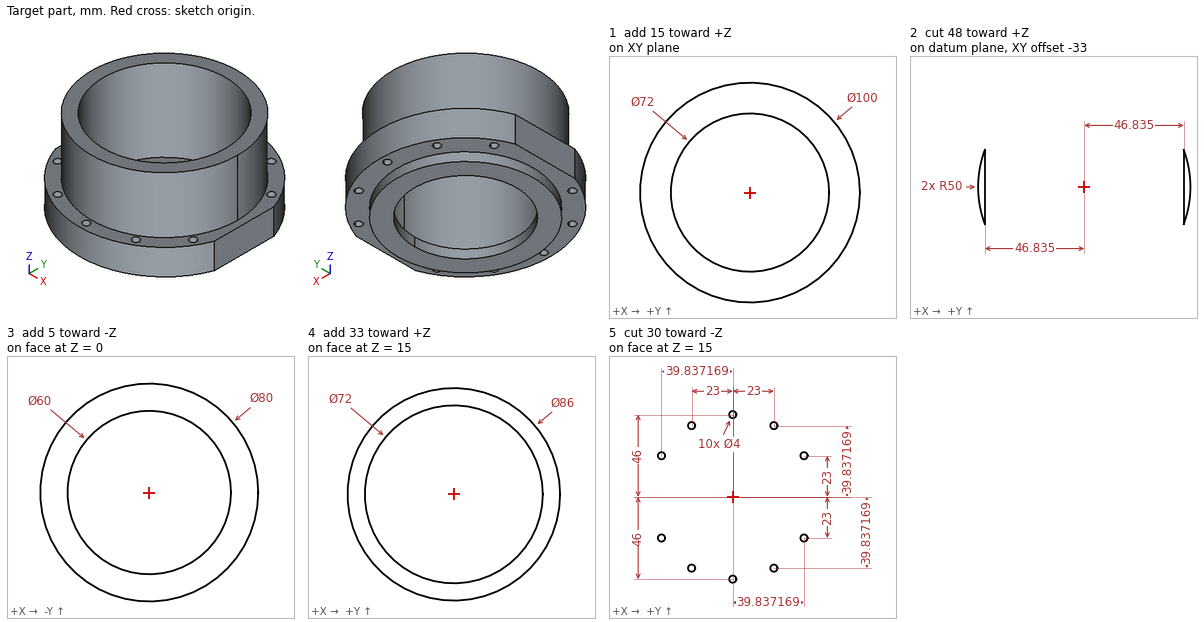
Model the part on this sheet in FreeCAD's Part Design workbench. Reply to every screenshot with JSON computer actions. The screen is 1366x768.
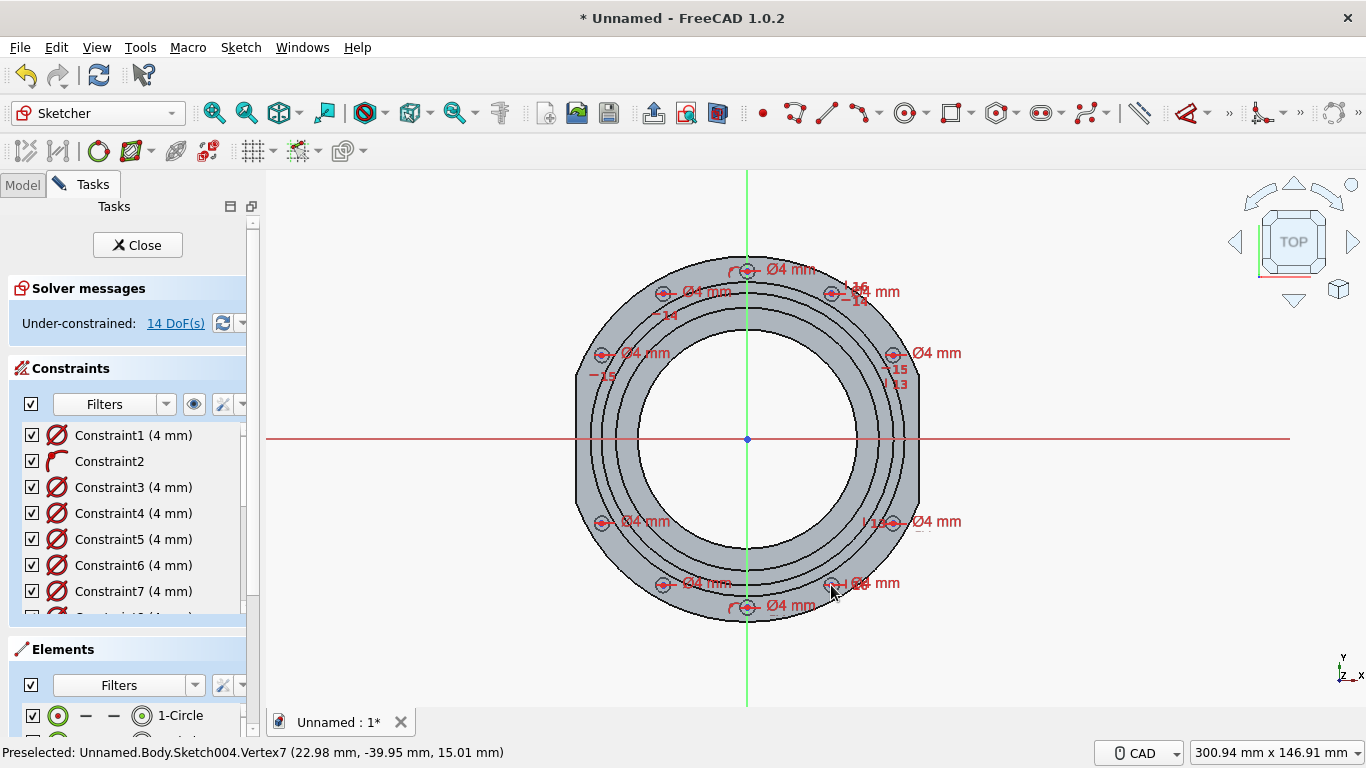
{"action": "left_click", "coordinate": [663, 294]}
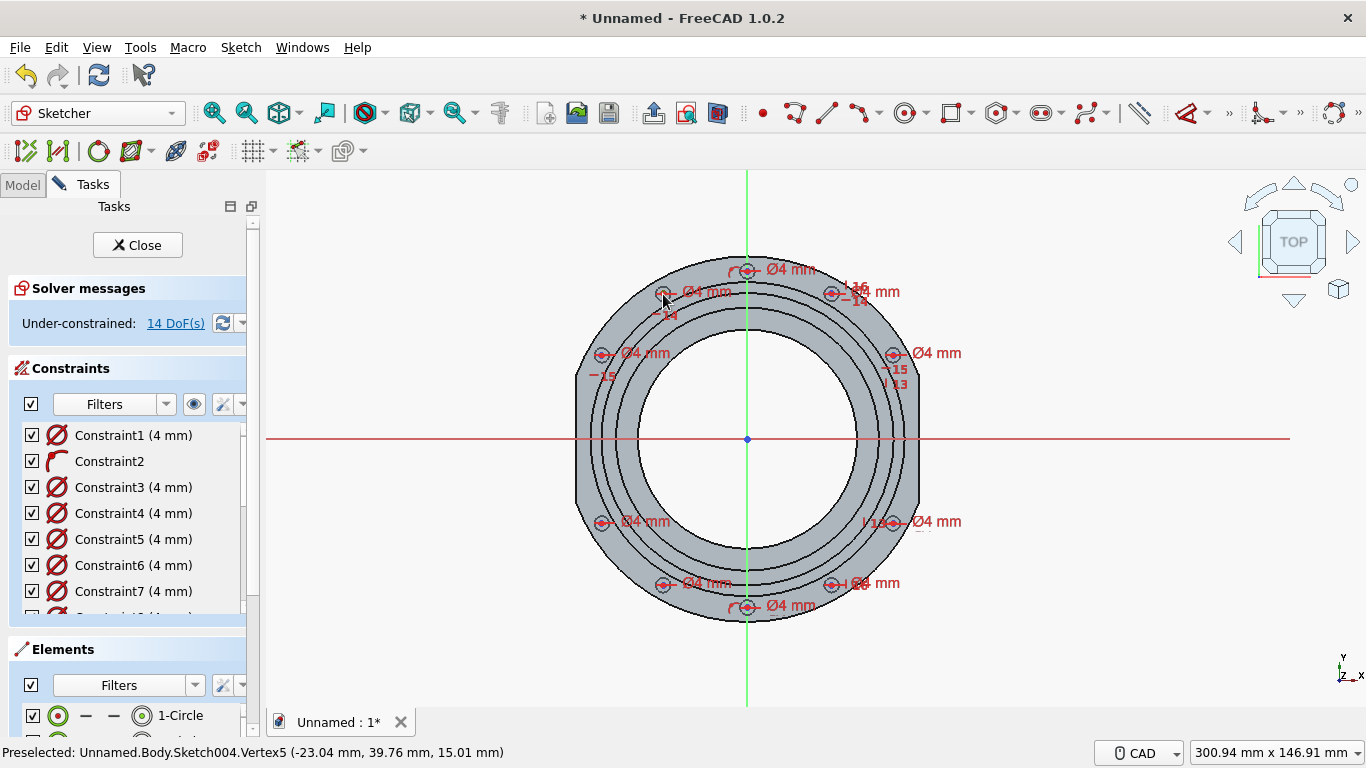
{"action": "left_click", "coordinate": [663, 585]}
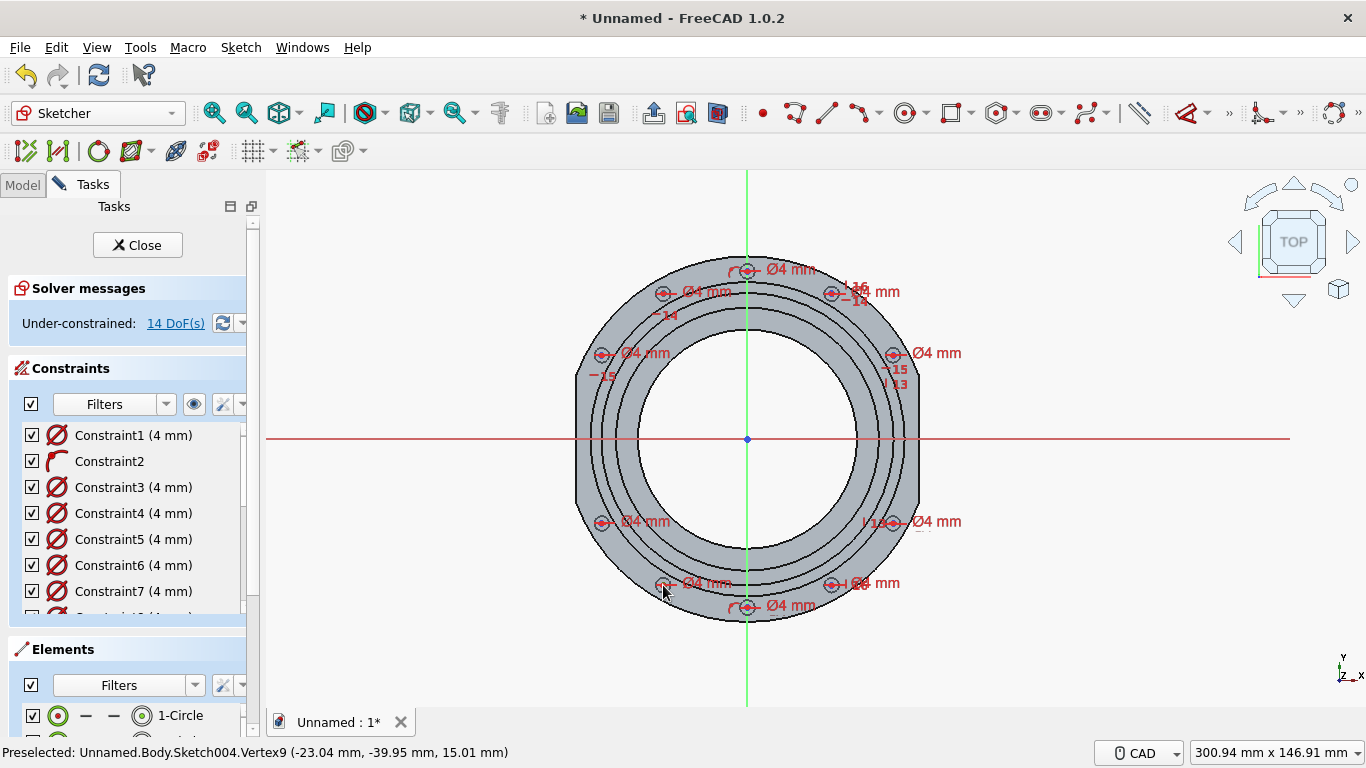
{"action": "key", "text": "v"}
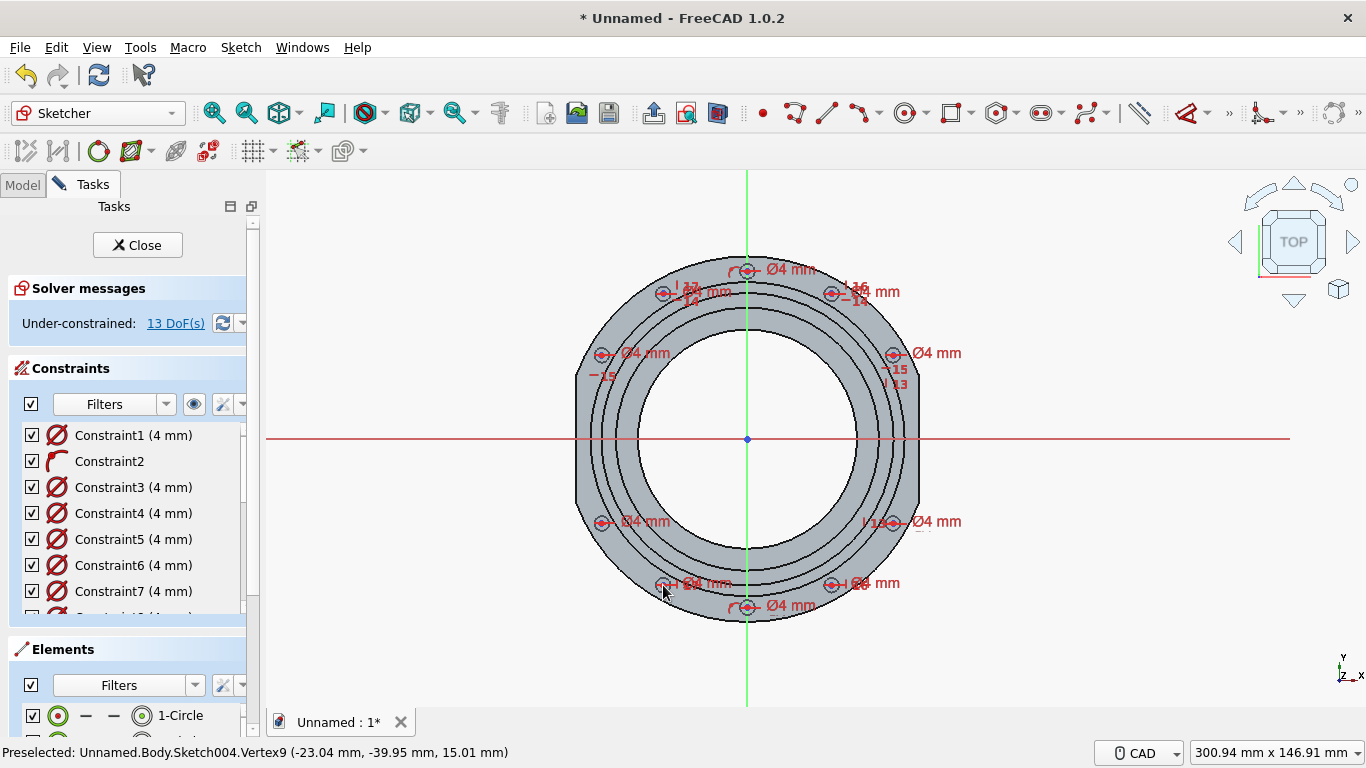
{"action": "left_click", "coordinate": [832, 585]}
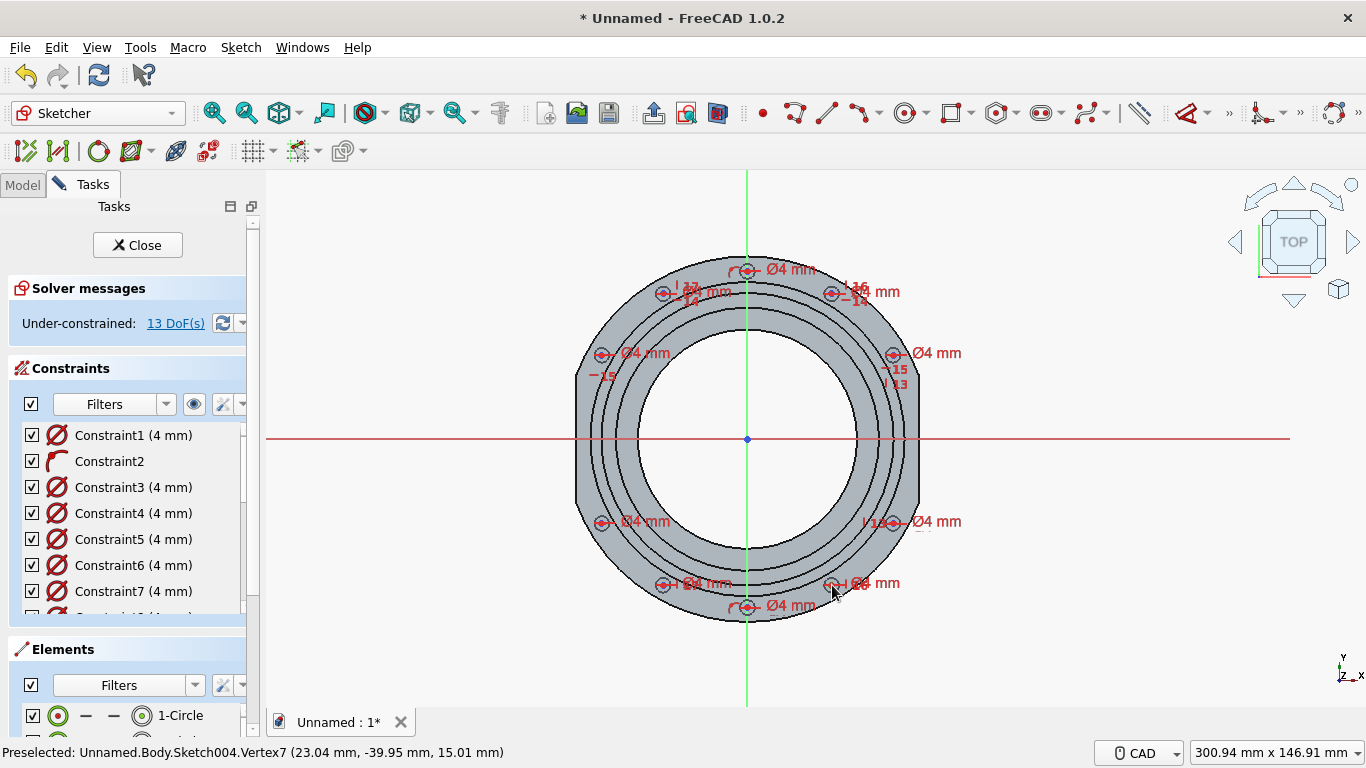
{"action": "left_click", "coordinate": [663, 585]}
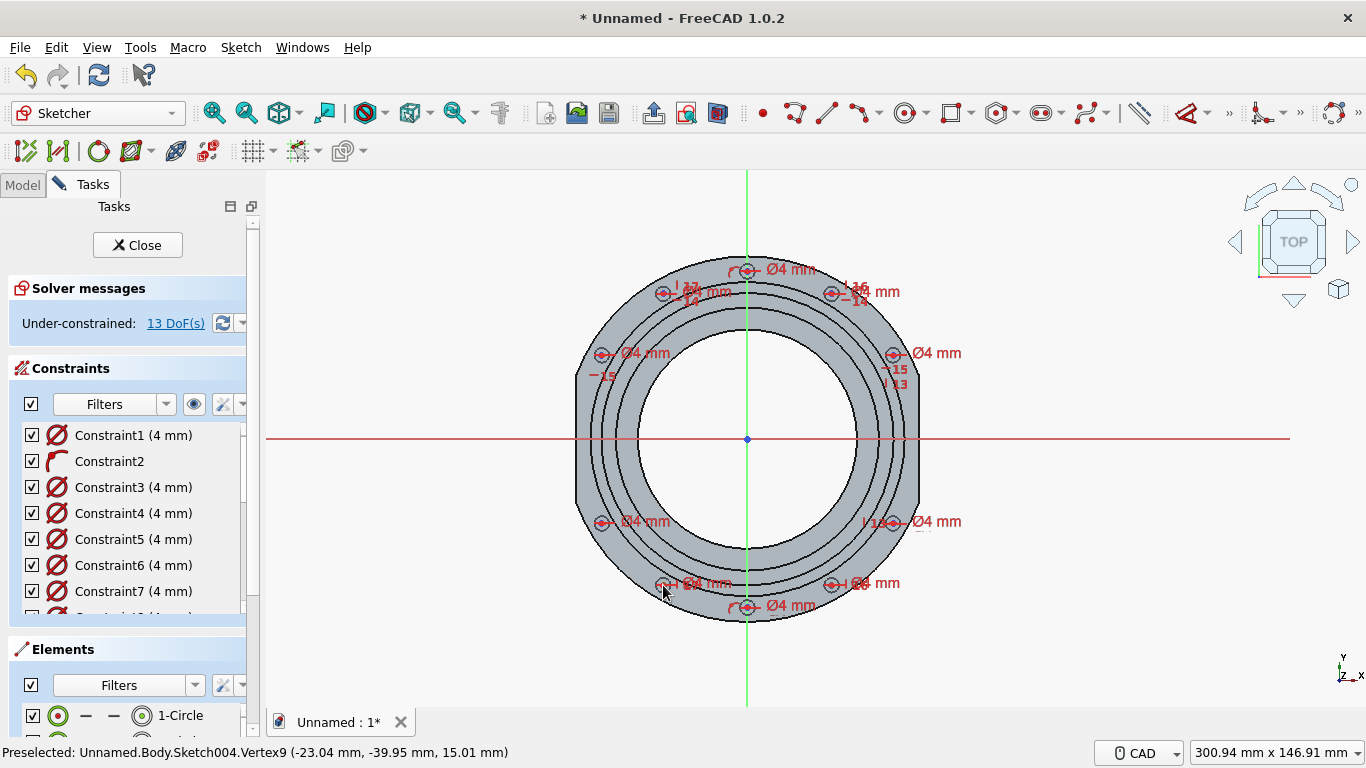
{"action": "key", "text": "h"}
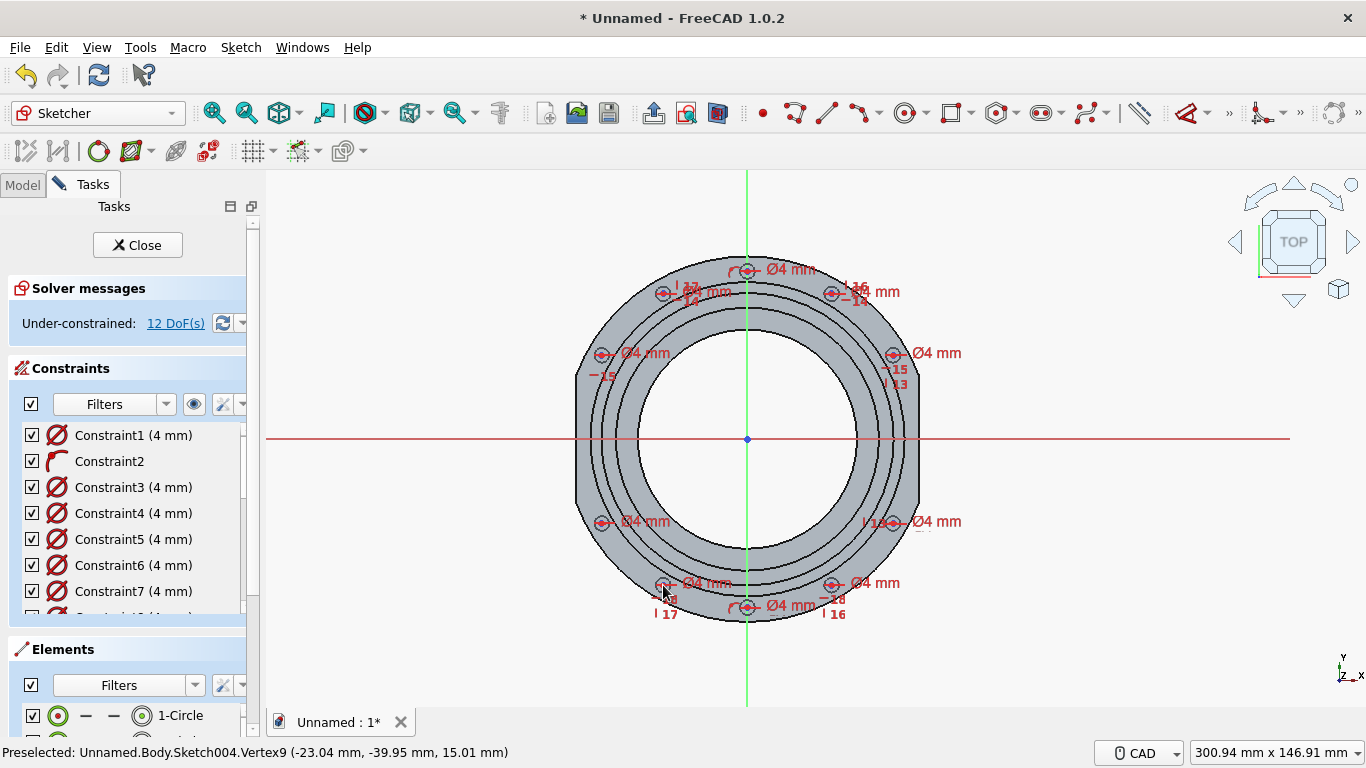
{"action": "left_click", "coordinate": [602, 355]}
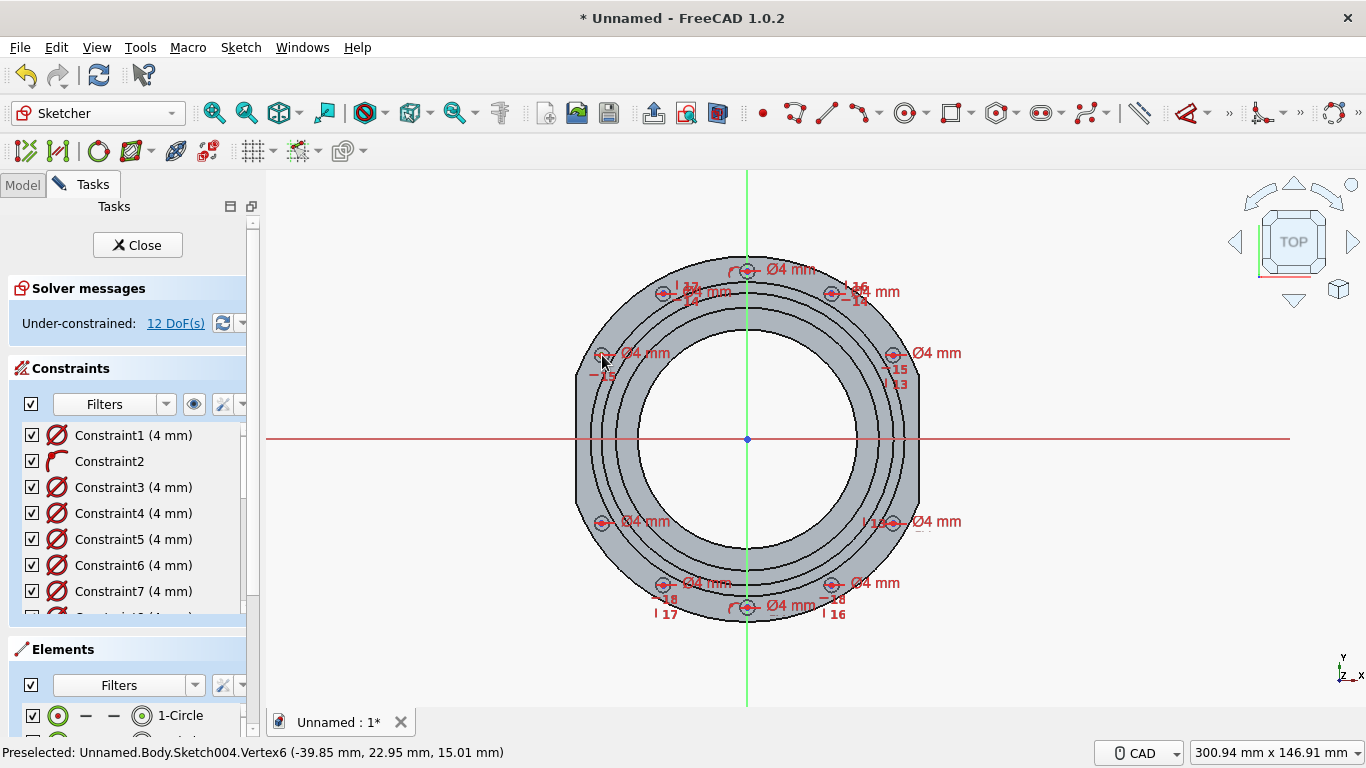
{"action": "left_click", "coordinate": [602, 523]}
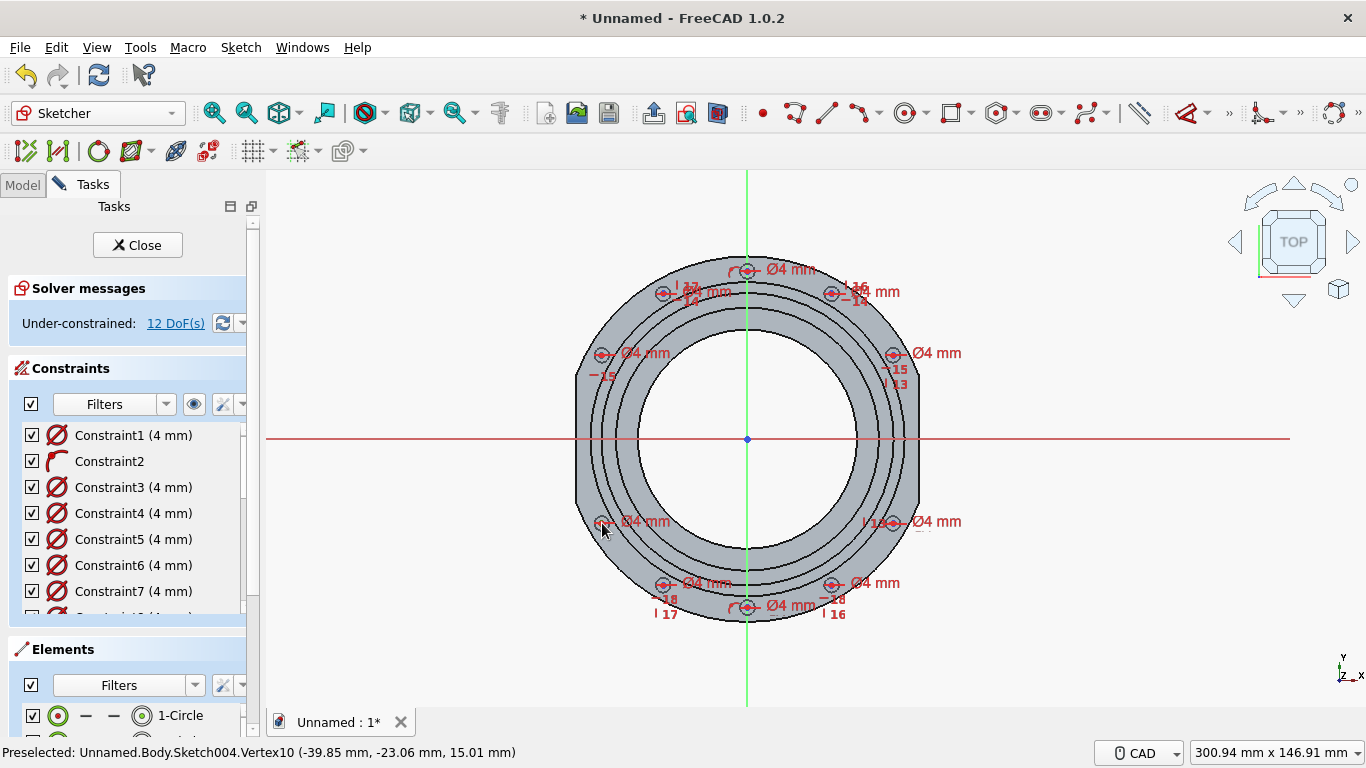
{"action": "key", "text": "v"}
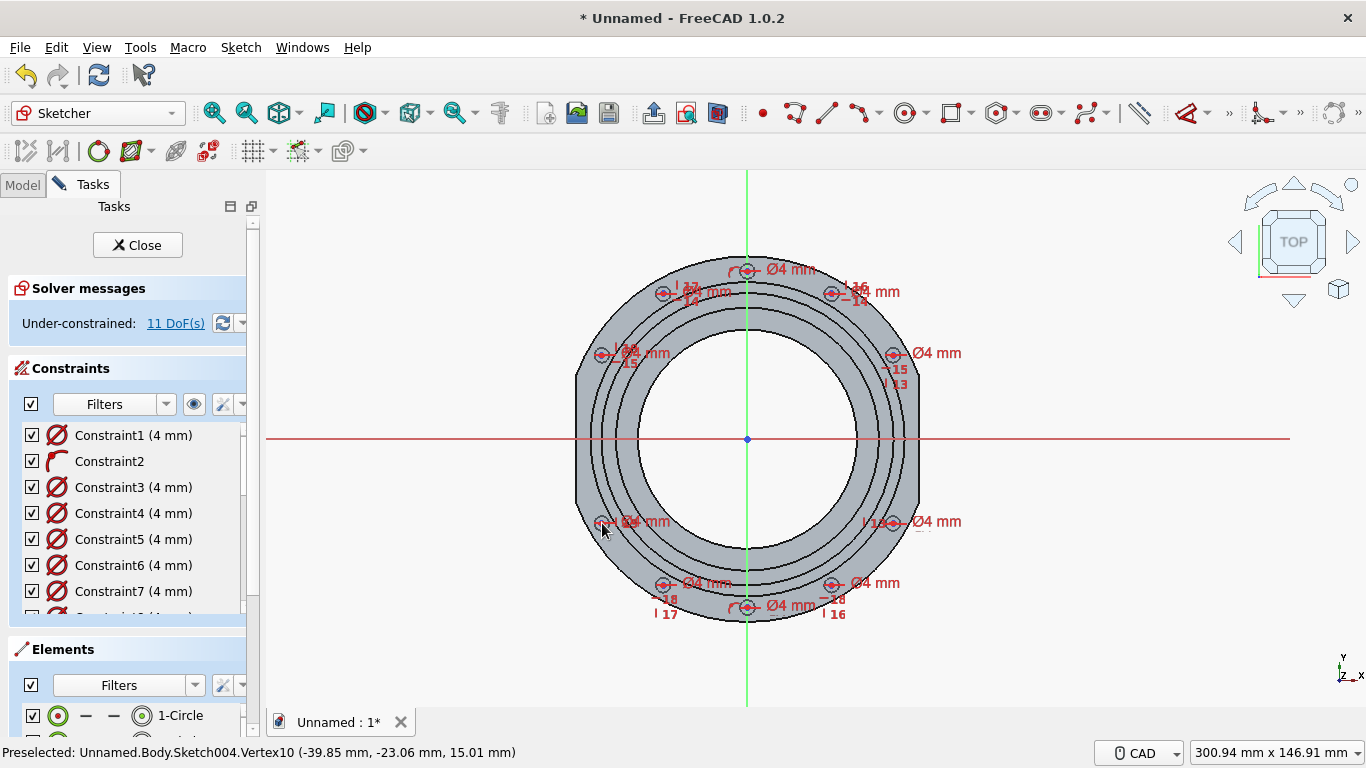
{"action": "left_click", "coordinate": [893, 524]}